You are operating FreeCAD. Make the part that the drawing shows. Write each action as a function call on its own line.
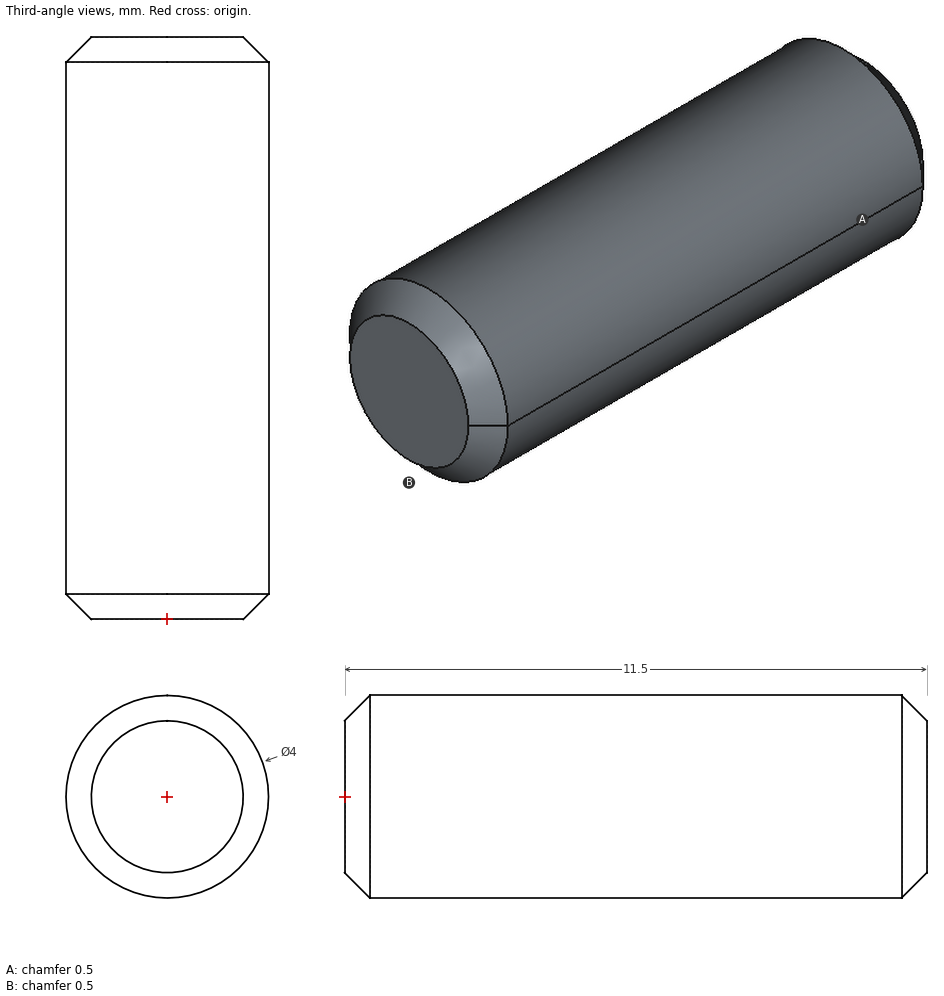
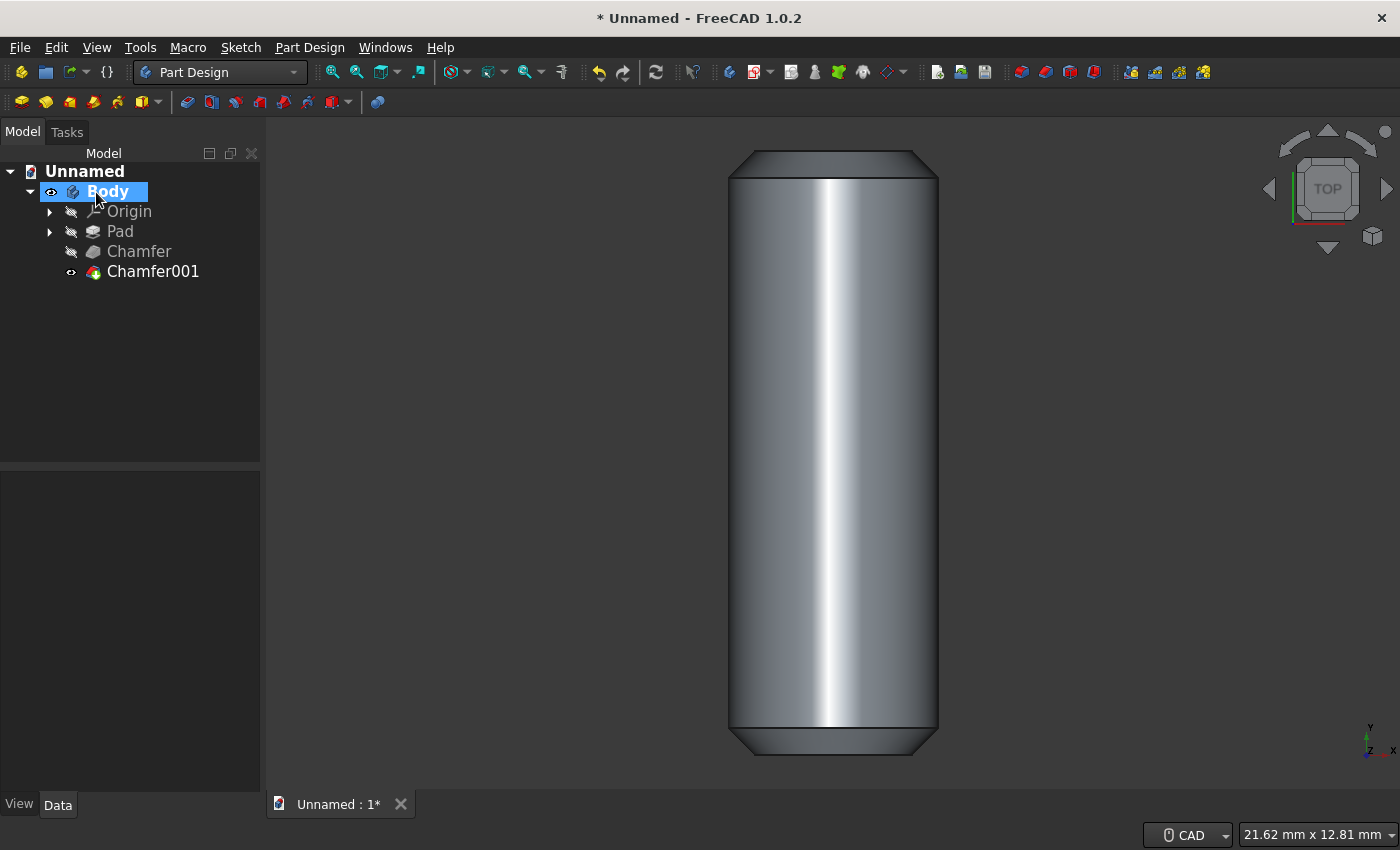
key(0)